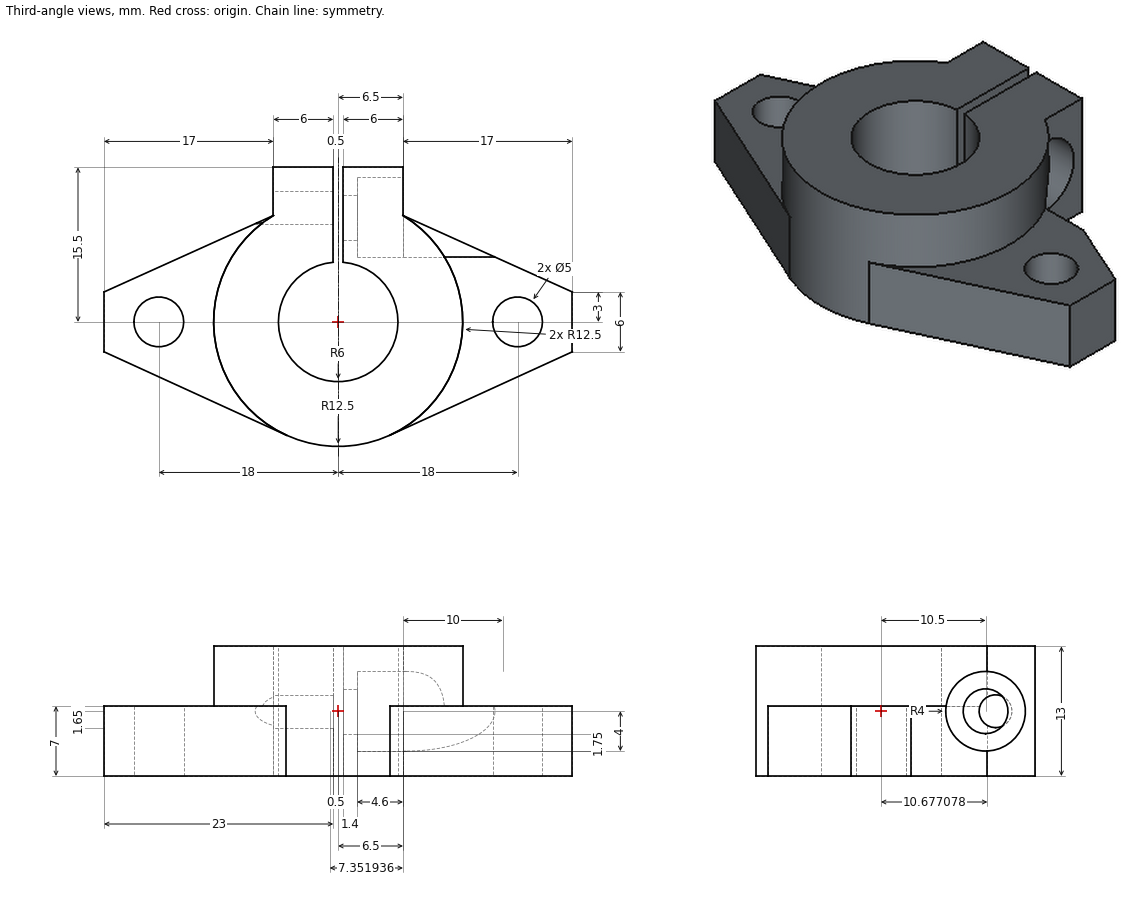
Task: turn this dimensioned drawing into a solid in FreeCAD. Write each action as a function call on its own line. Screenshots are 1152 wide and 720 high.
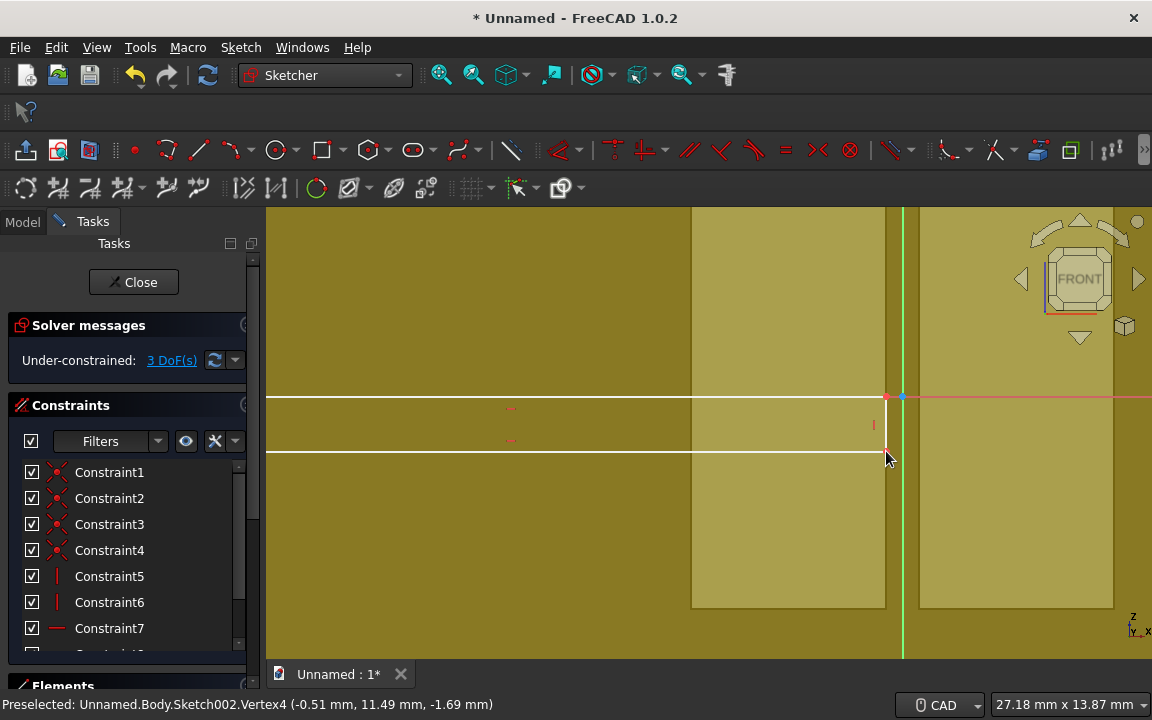
click(558, 150)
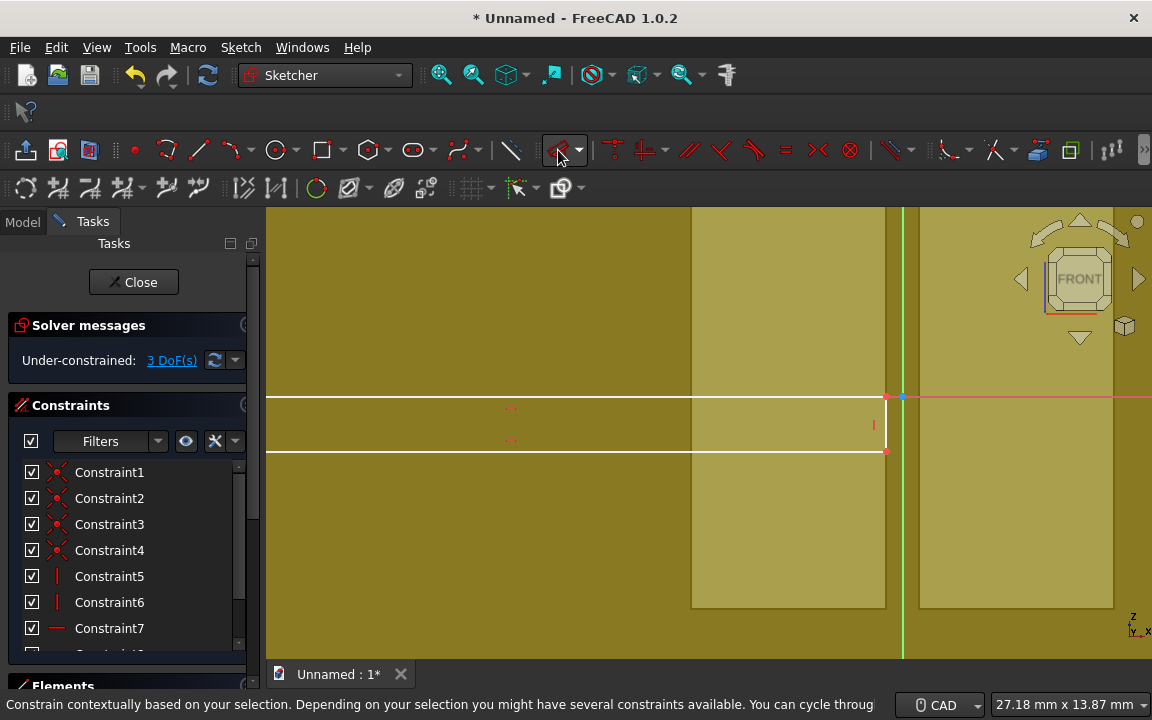
click(362, 452)
click(590, 486)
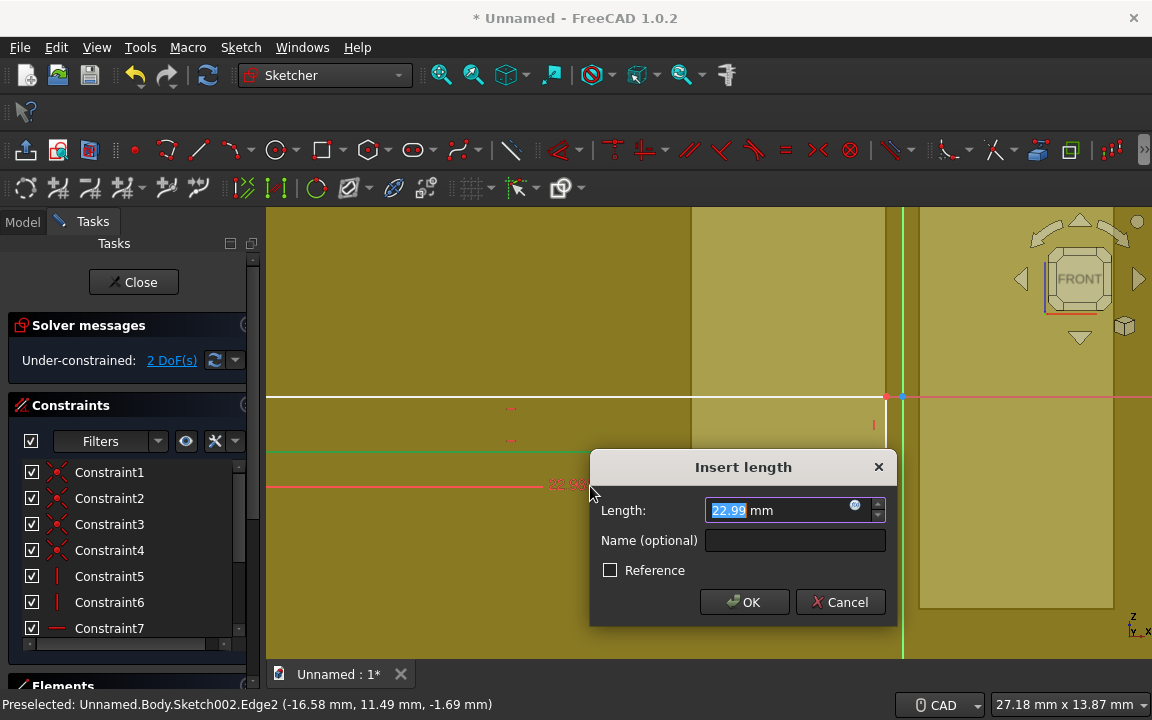
text(23)
key(Return)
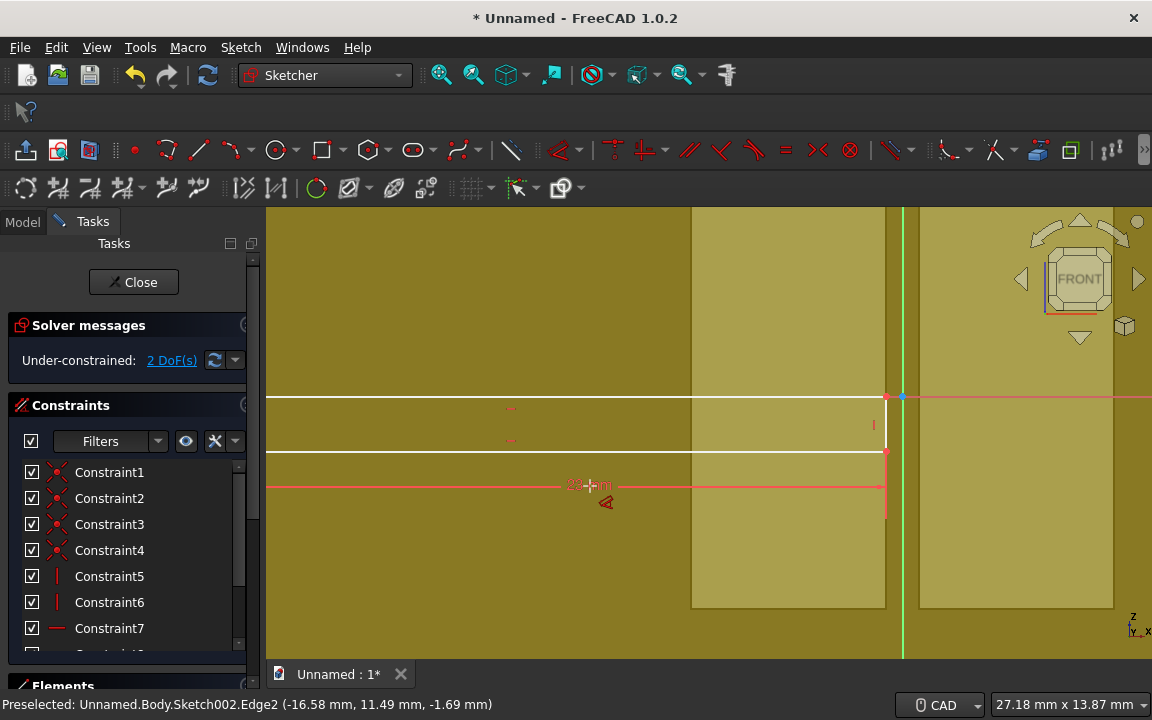
scroll(886, 452, down, 2)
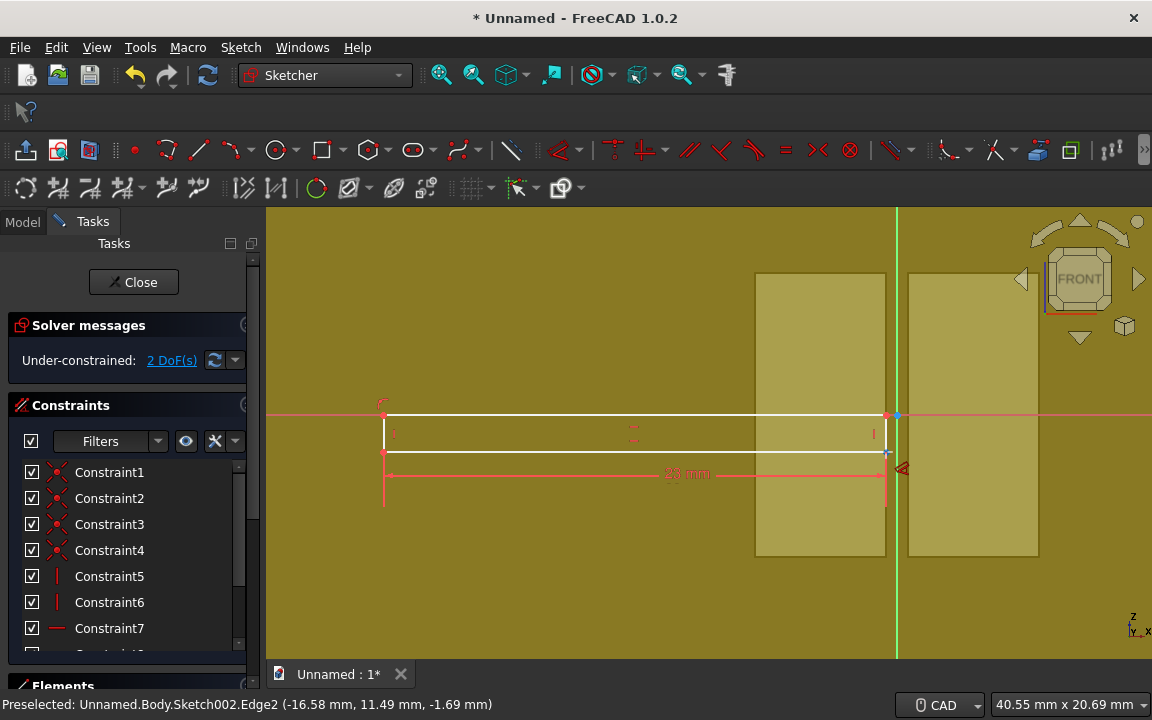
scroll(384, 426, up, 2)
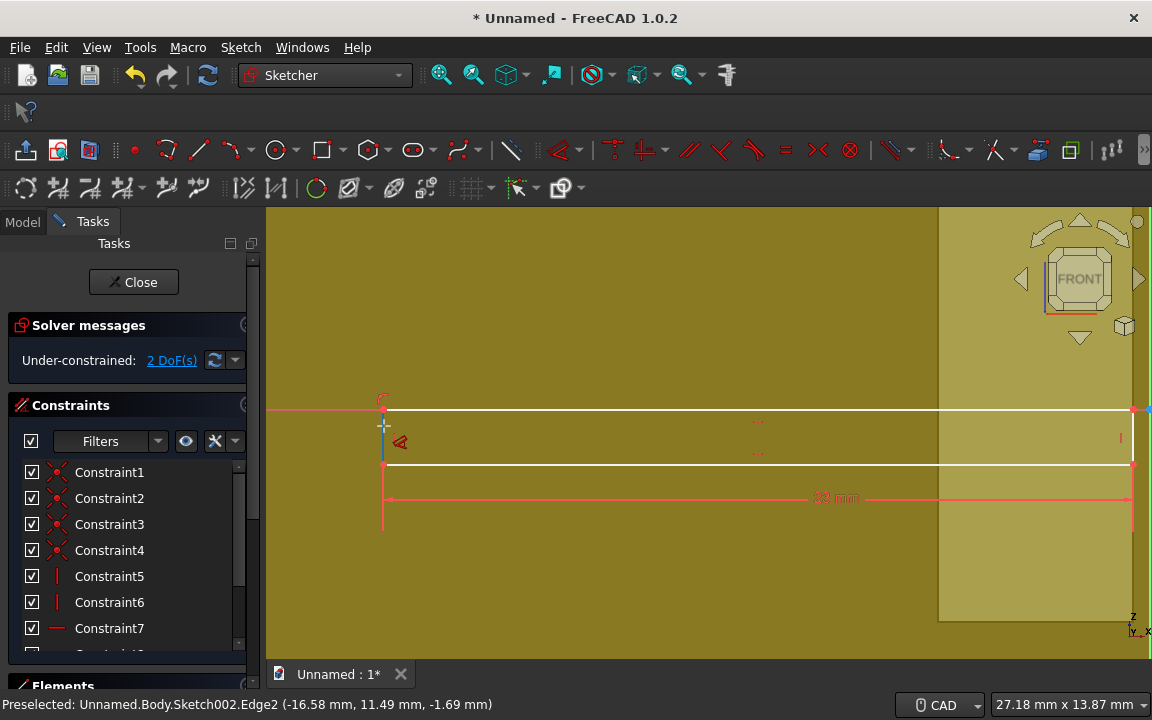
click(383, 426)
click(349, 437)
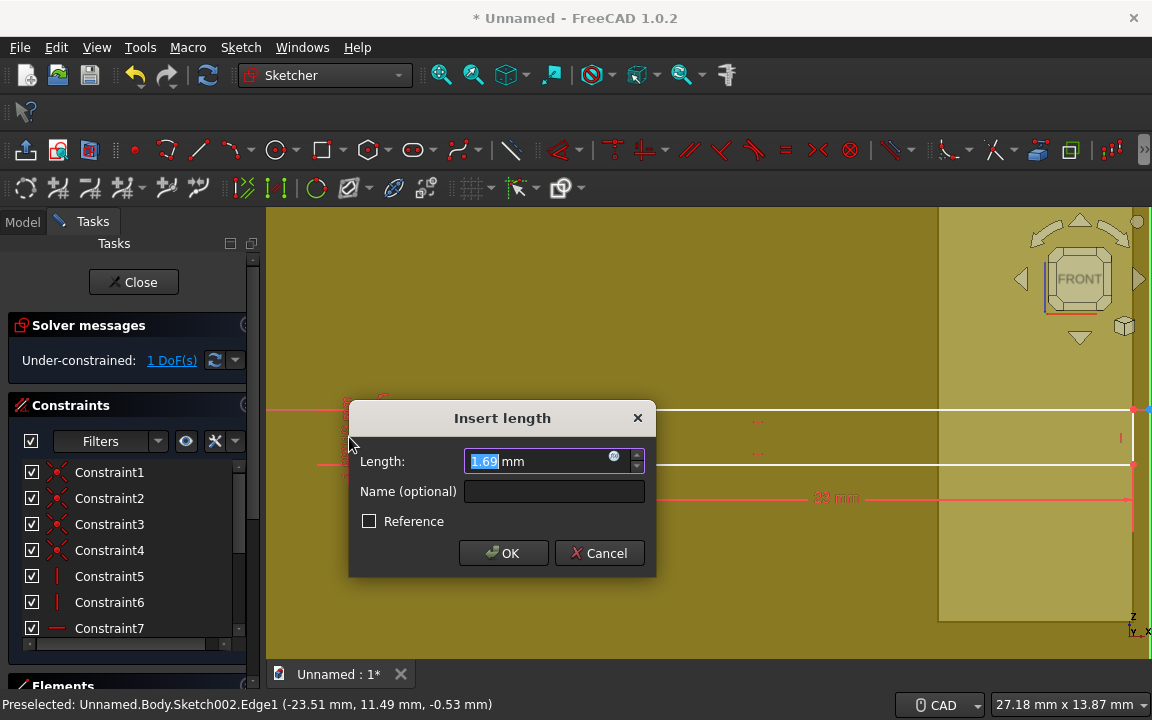
text(1.65)
key(Return)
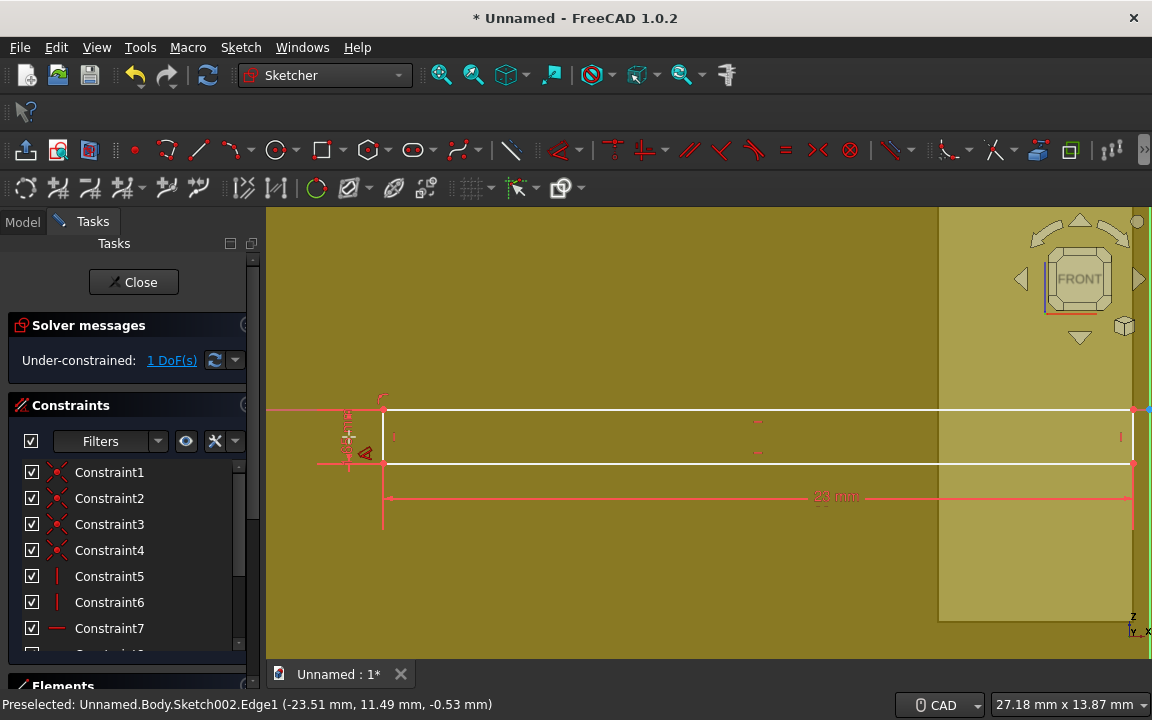
scroll(384, 426, down, 2)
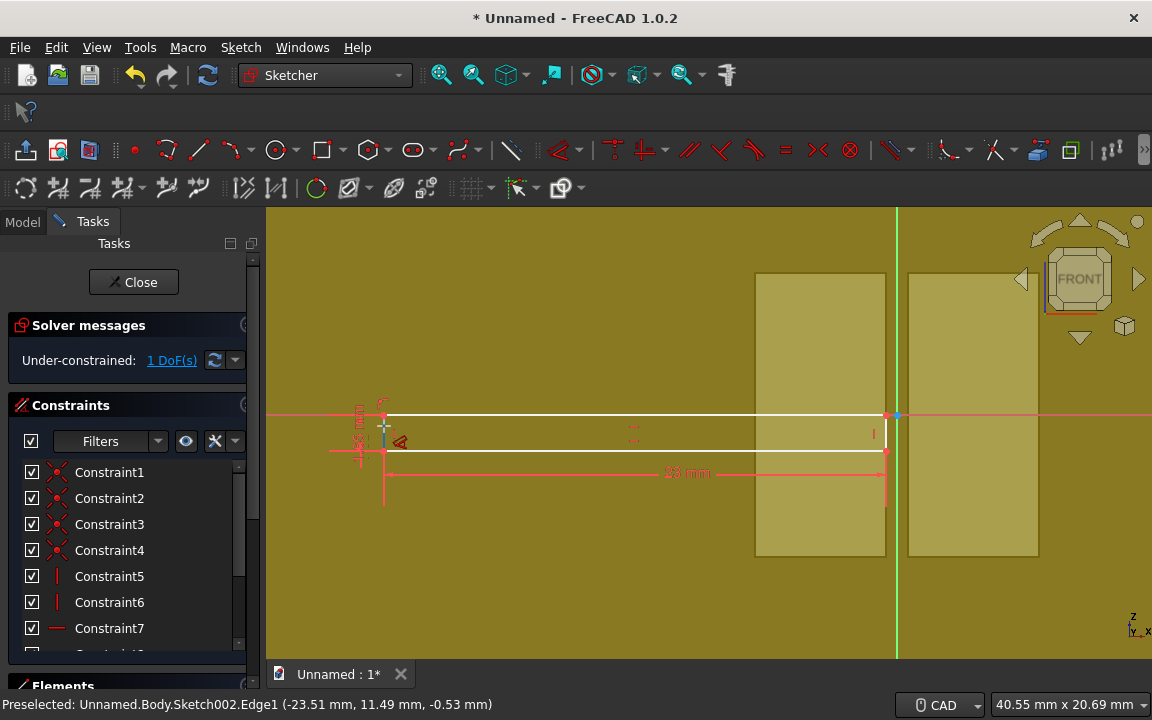
scroll(886, 451, up, 7)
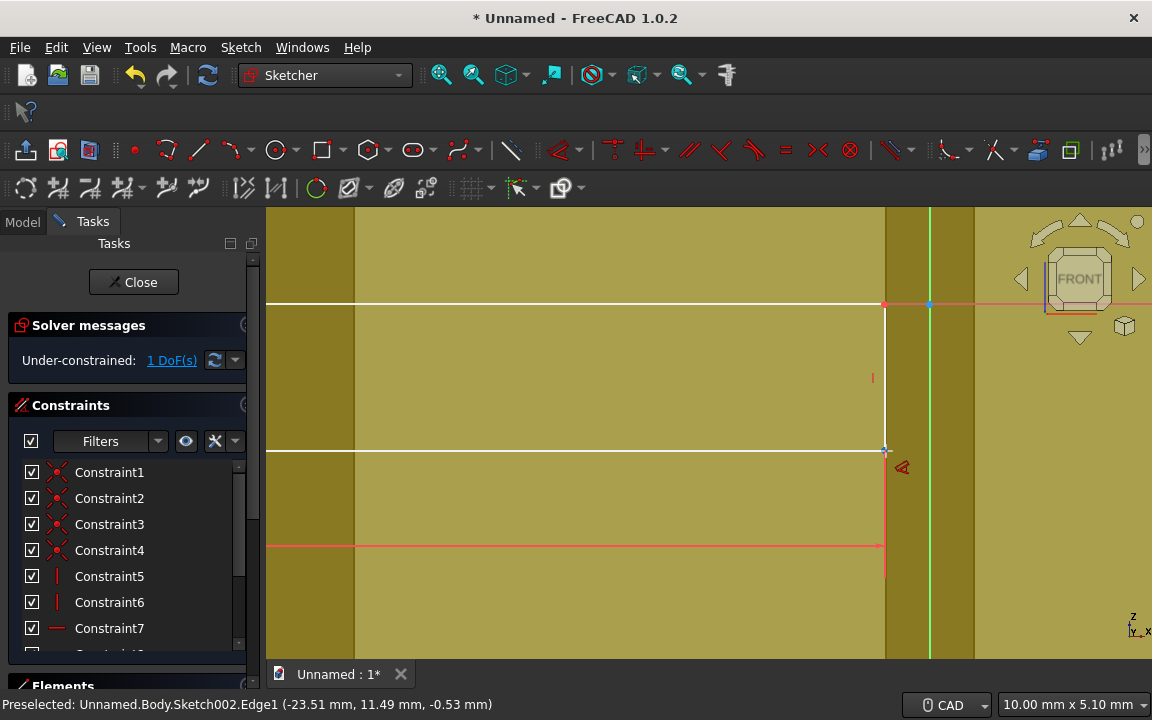
click(885, 451)
click(907, 485)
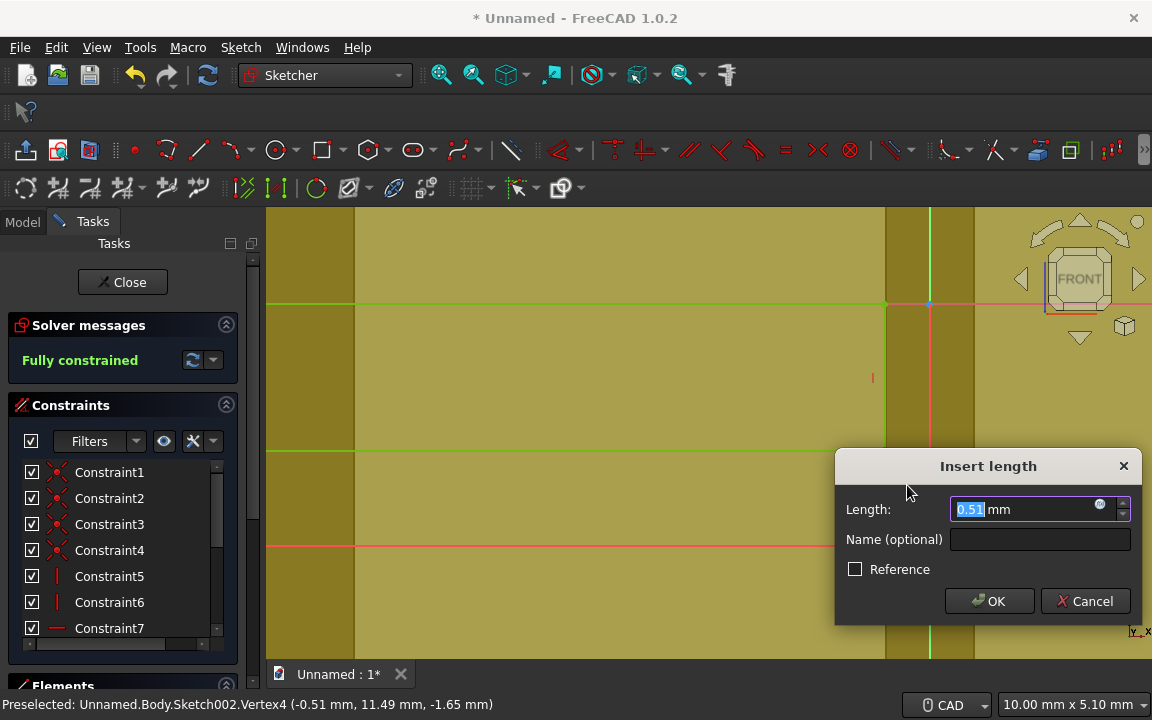
text(0.5)
key(Return)
key(Escape)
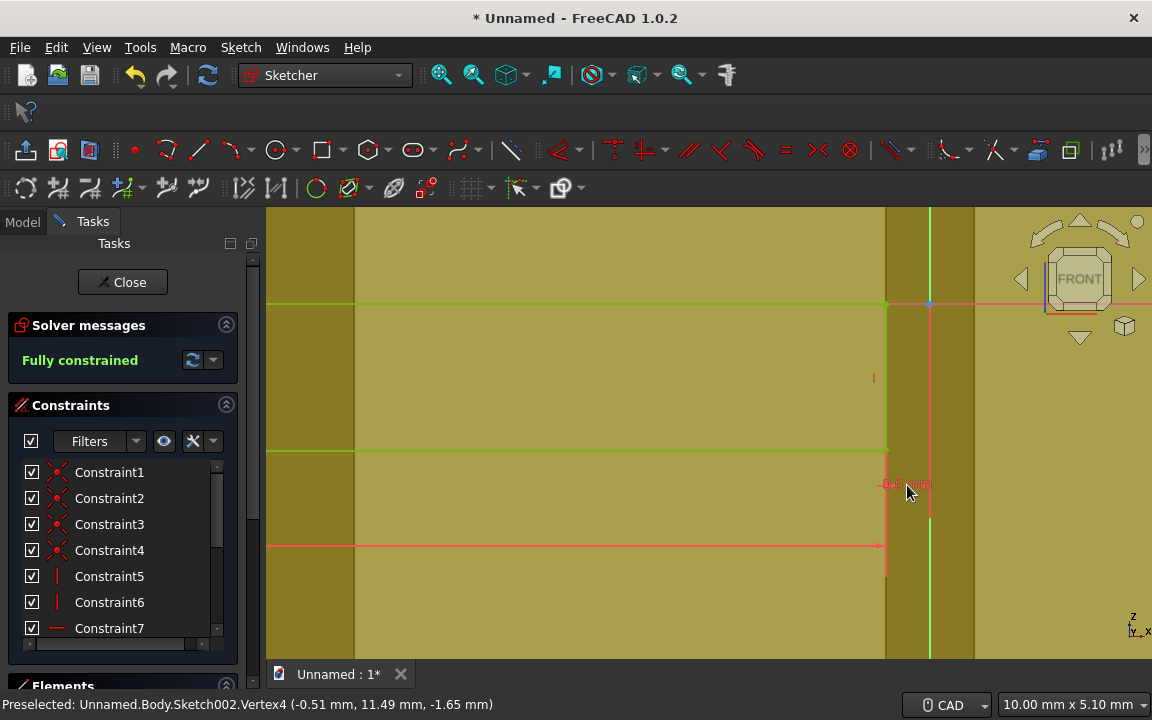
click(123, 282)